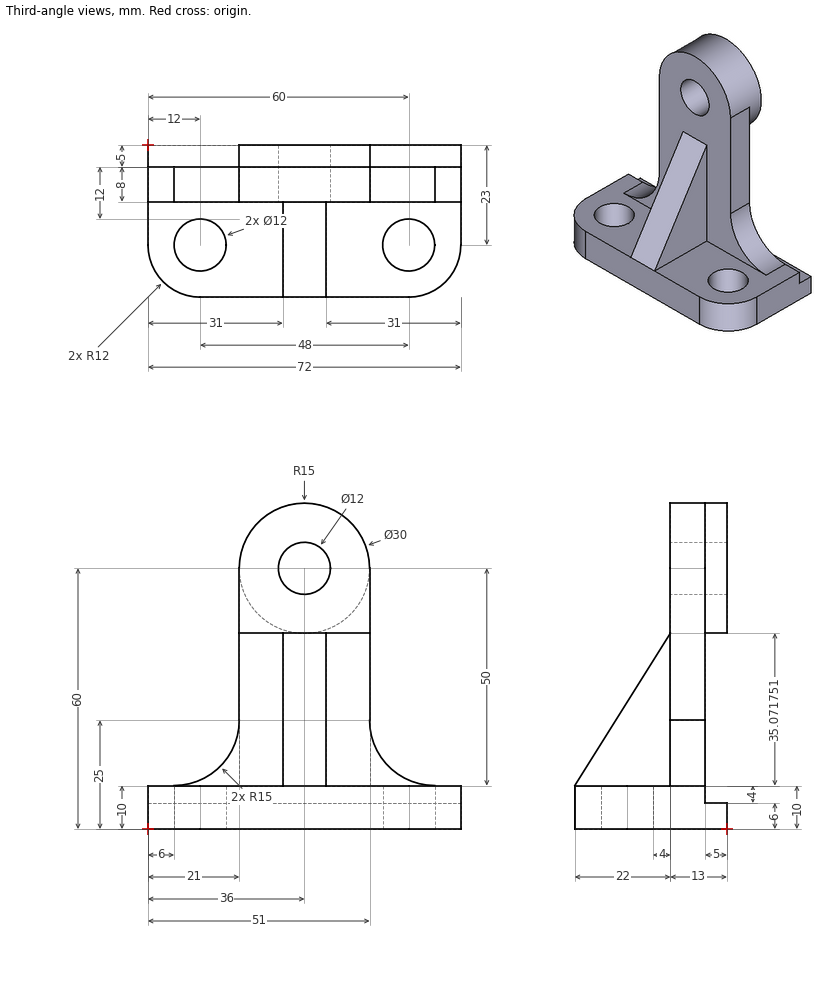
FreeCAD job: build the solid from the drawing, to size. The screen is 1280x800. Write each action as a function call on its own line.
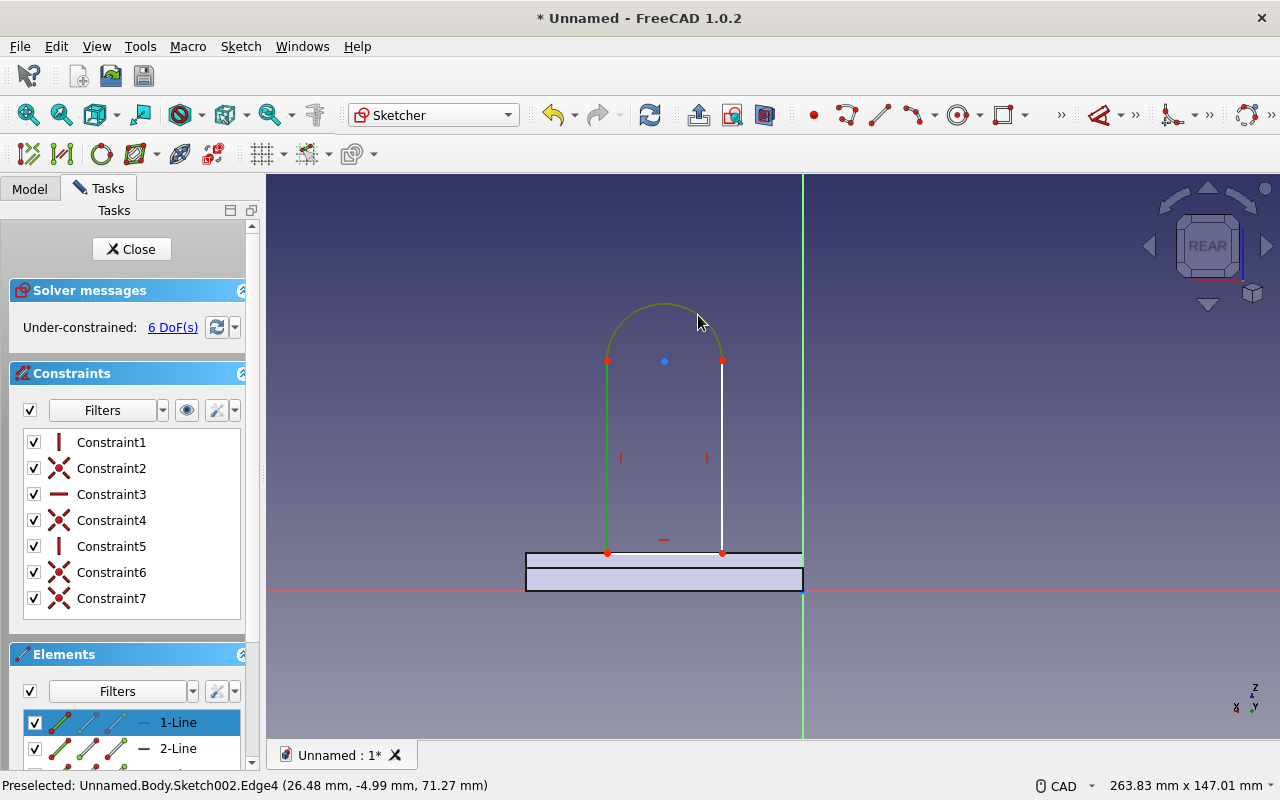
key(t)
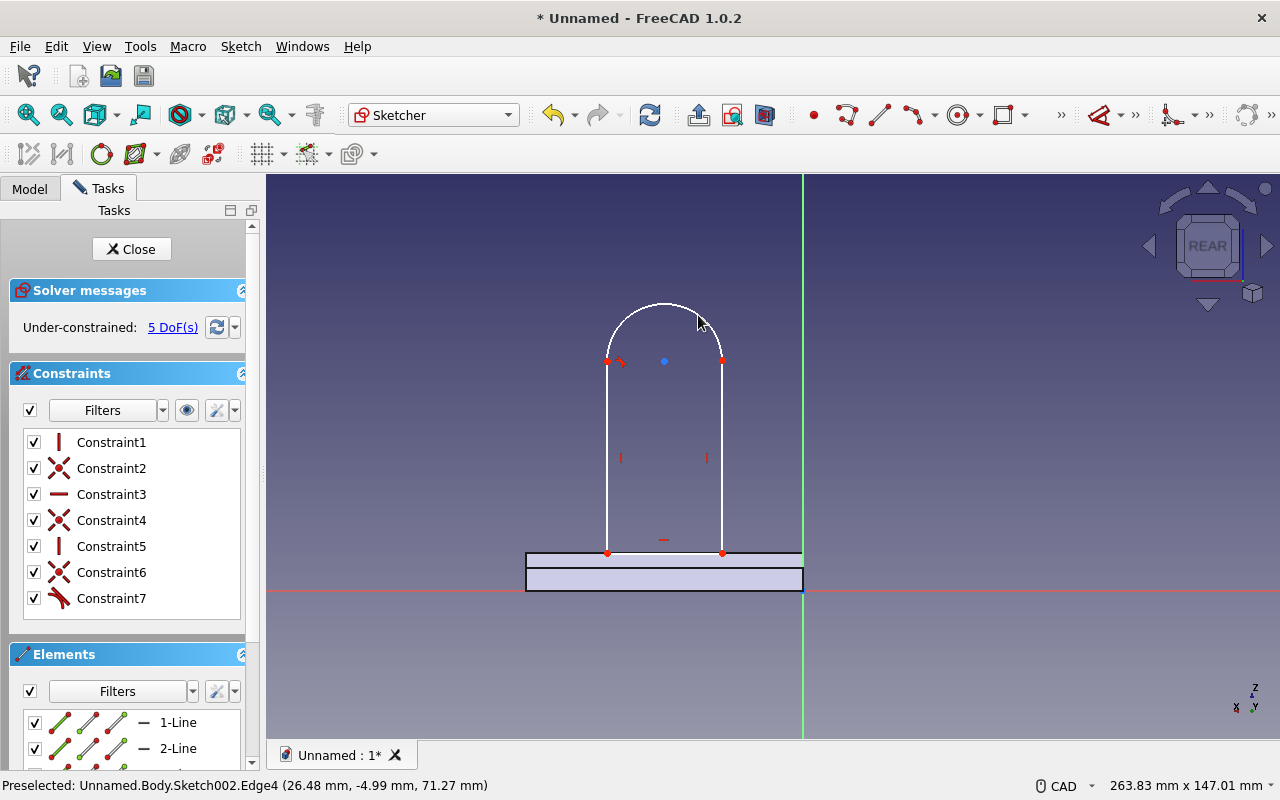
click(722, 496)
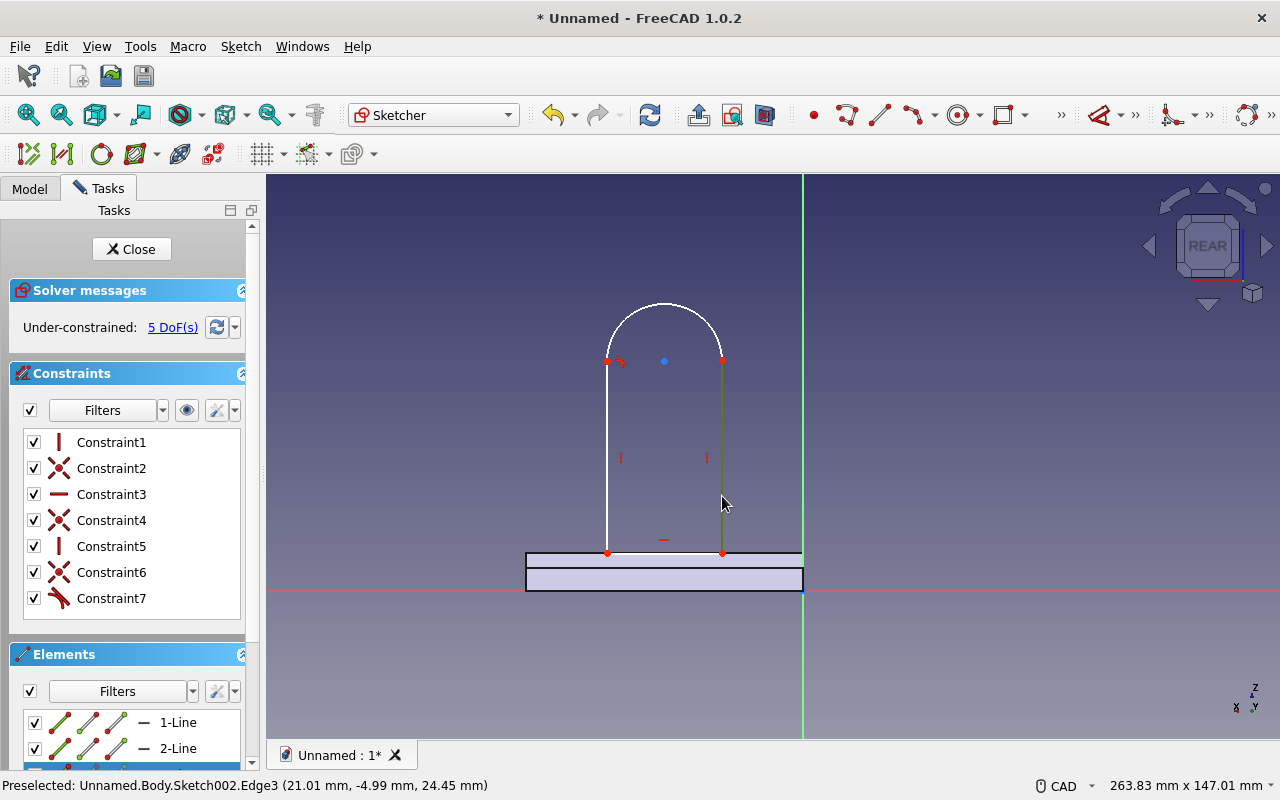
click(698, 315)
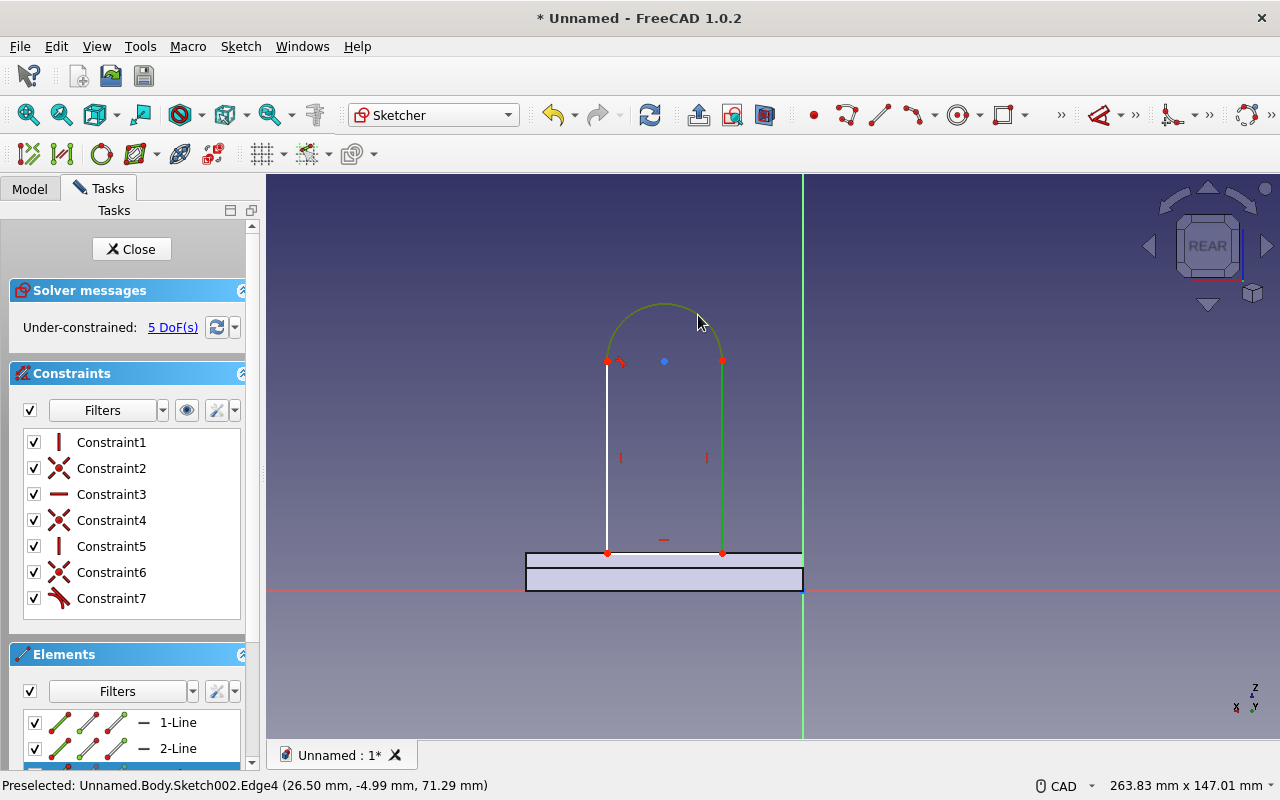
key(t)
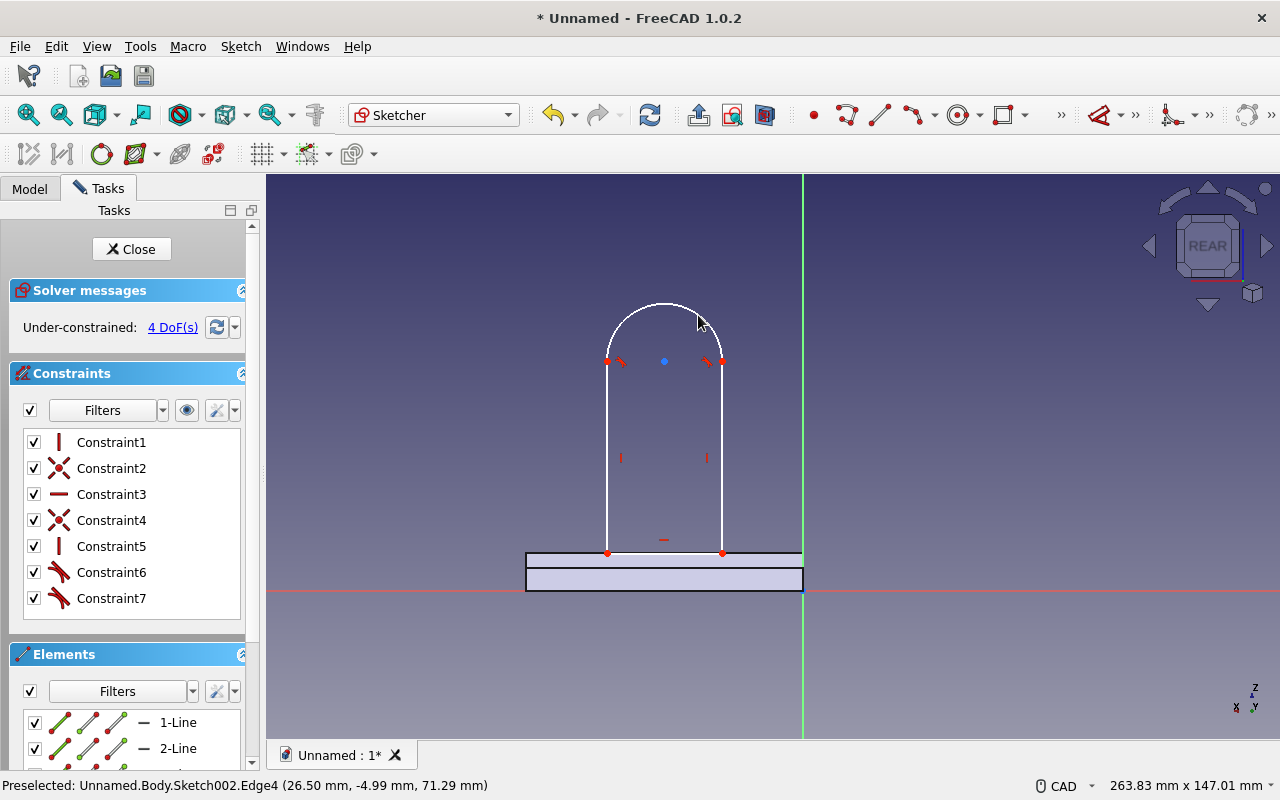
click(1098, 116)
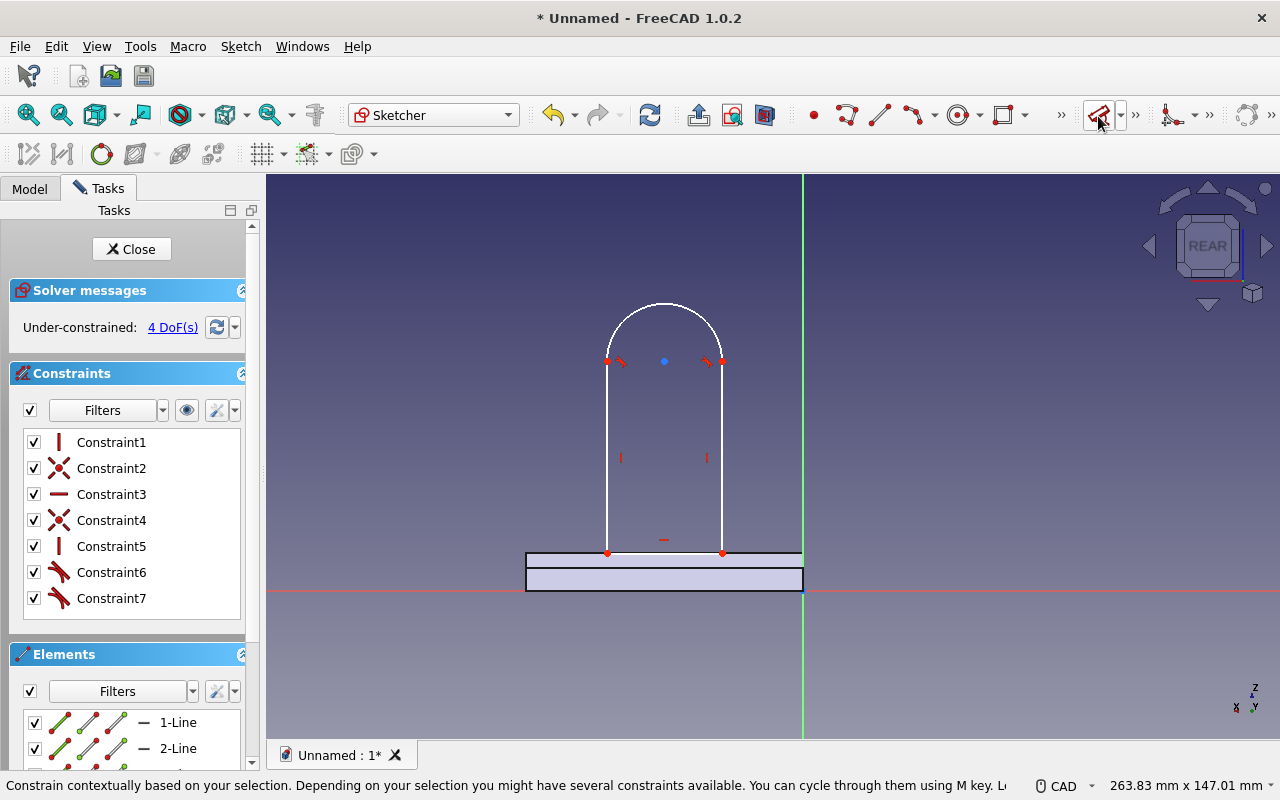
click(698, 315)
click(717, 289)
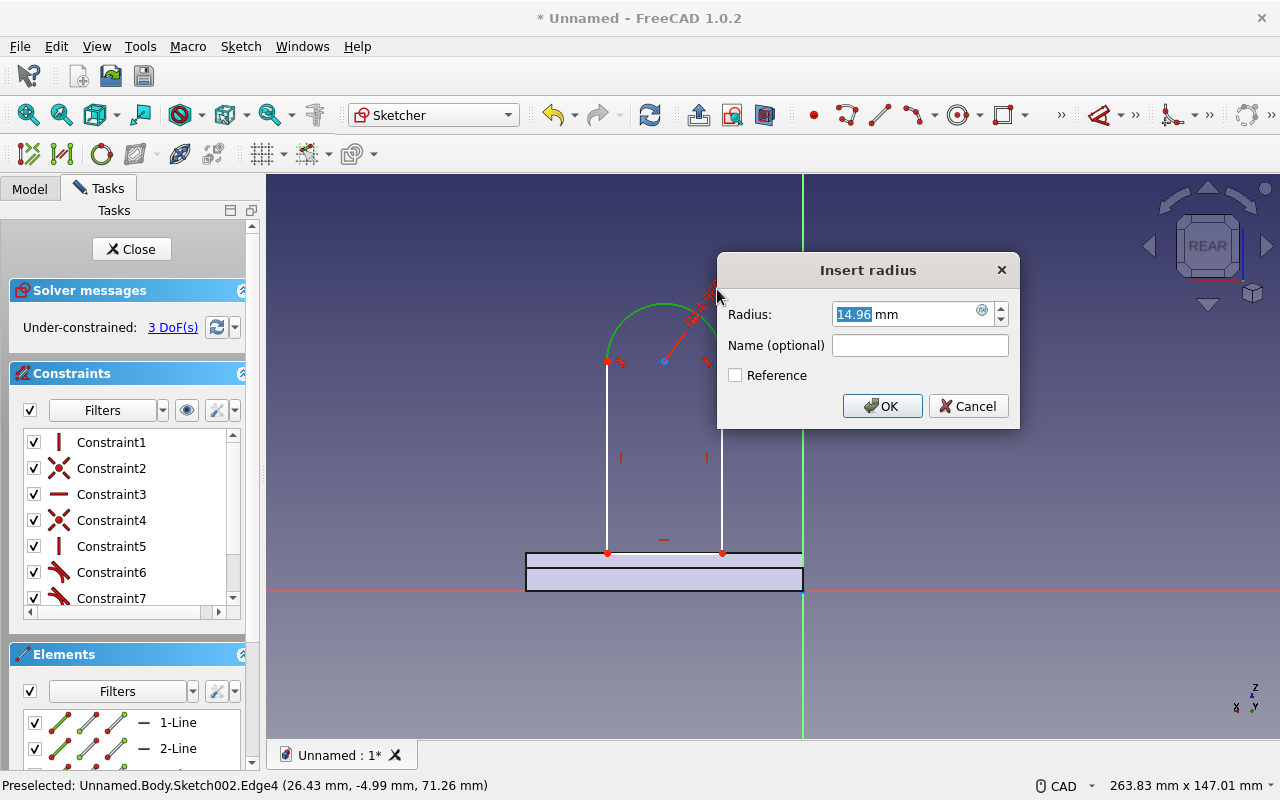
text(15)
key(Return)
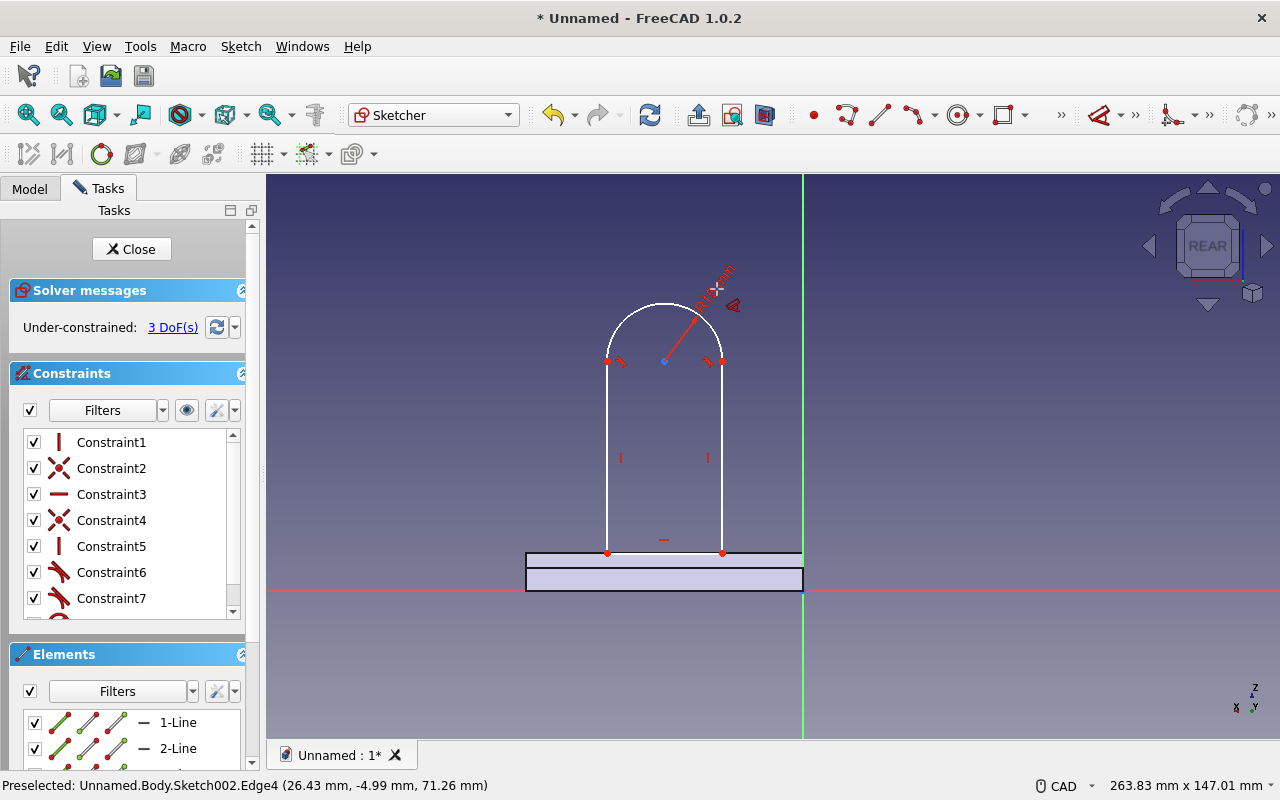
click(607, 419)
click(573, 458)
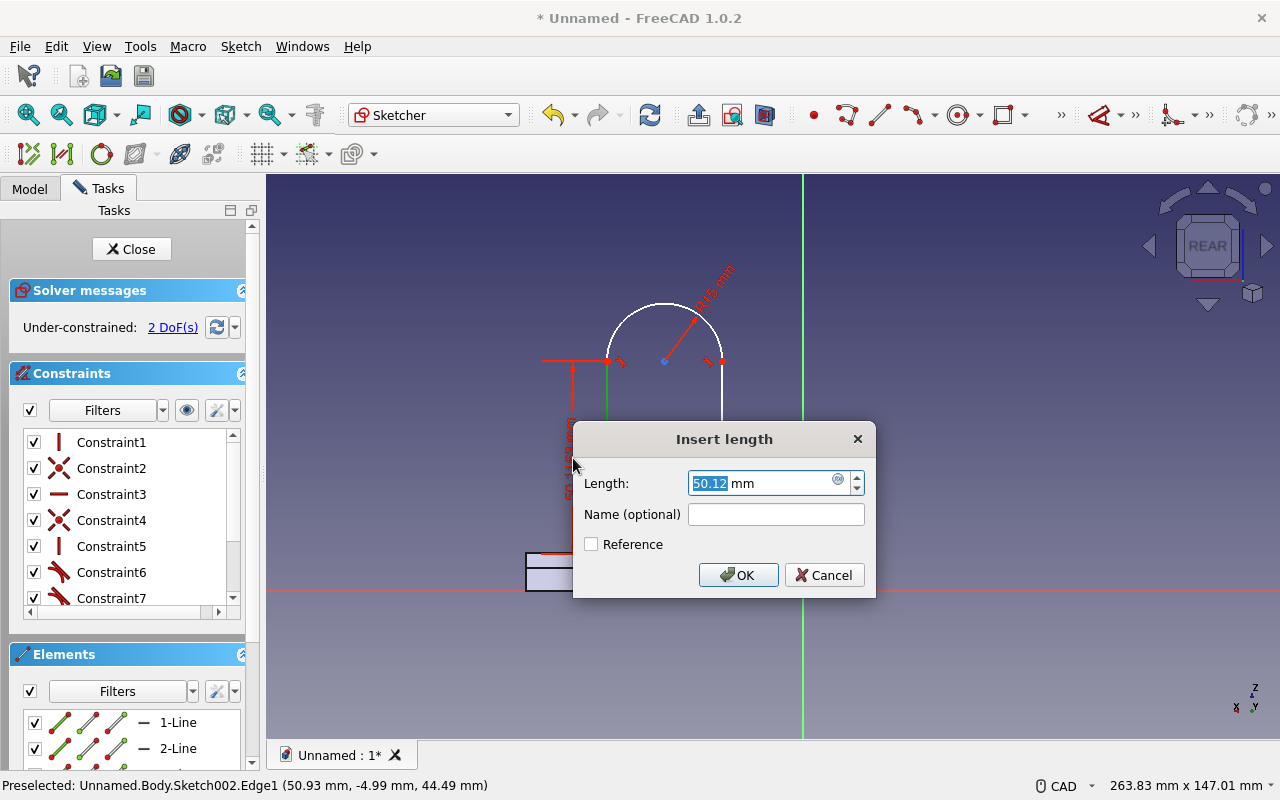
text(50)
key(Return)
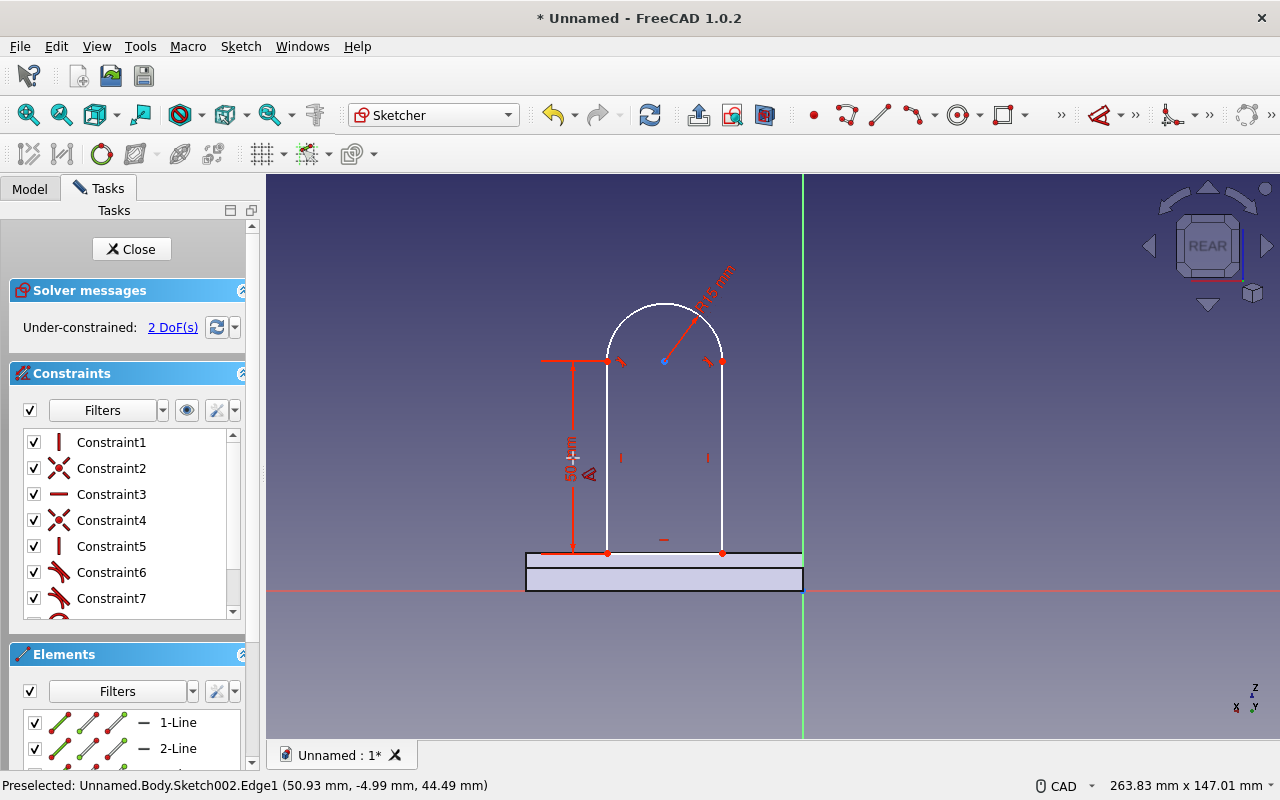
click(607, 361)
click(705, 625)